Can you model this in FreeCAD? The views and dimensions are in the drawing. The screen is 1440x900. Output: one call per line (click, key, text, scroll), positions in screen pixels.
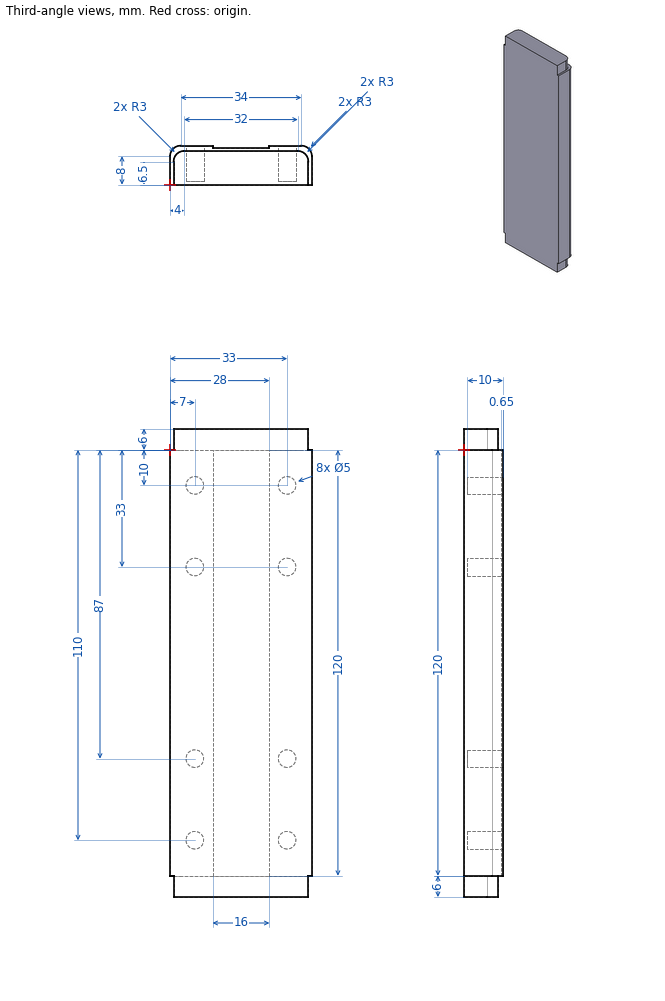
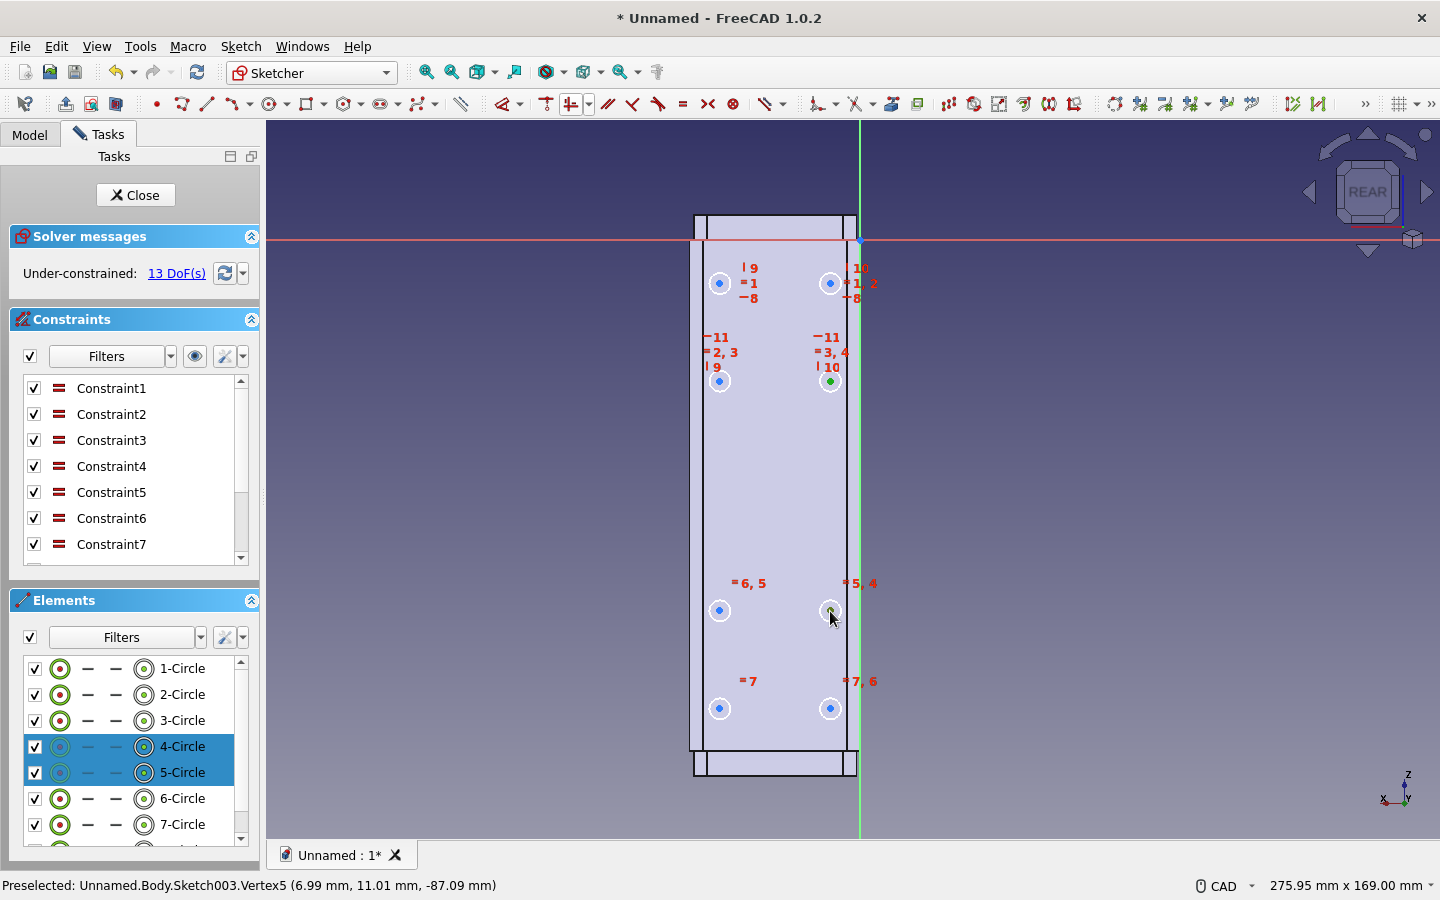
click(588, 104)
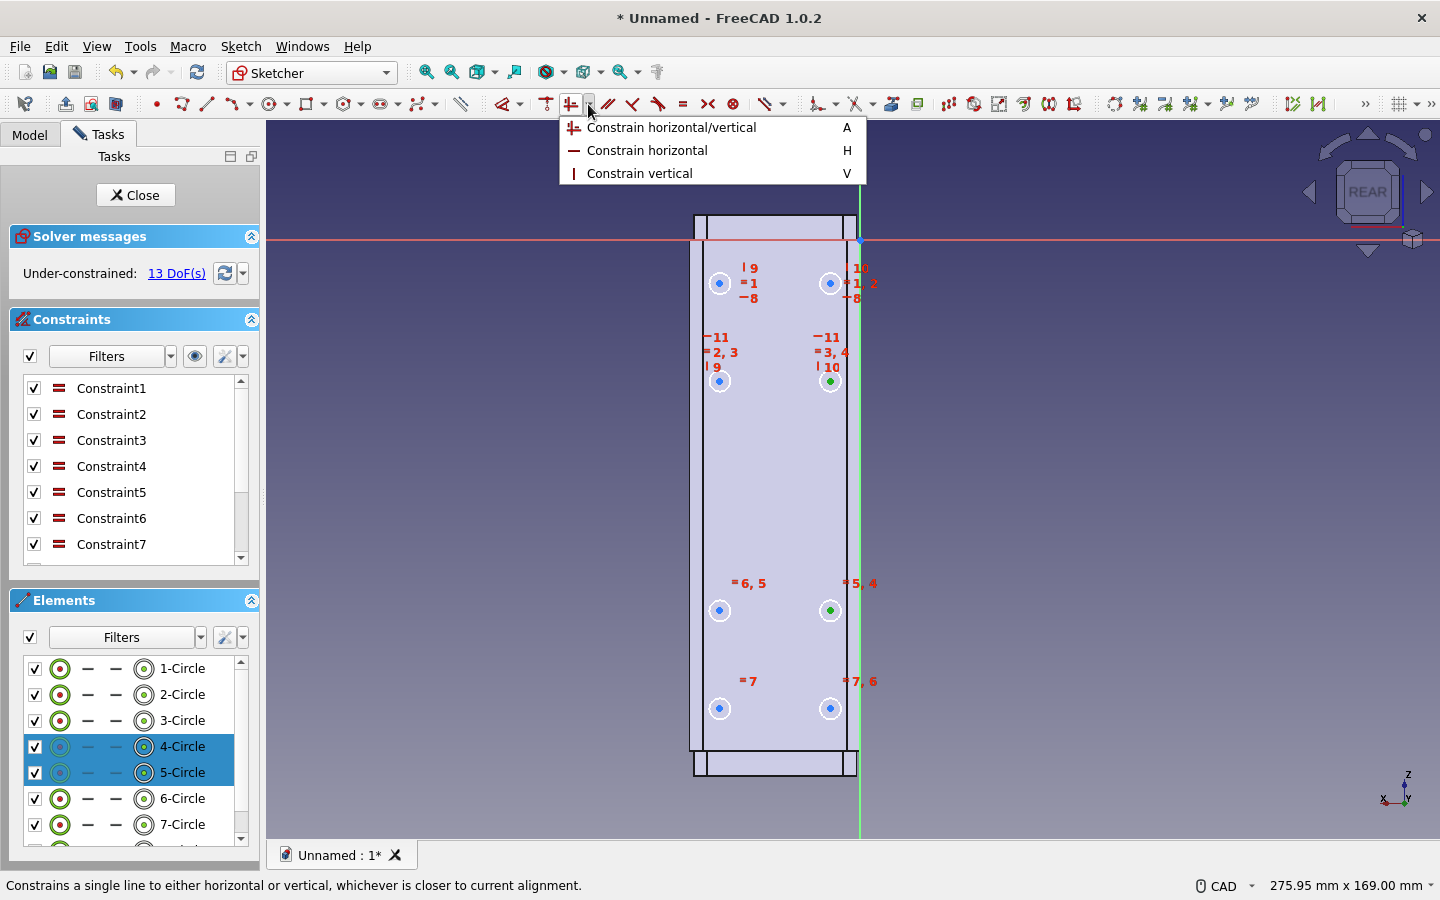
click(713, 174)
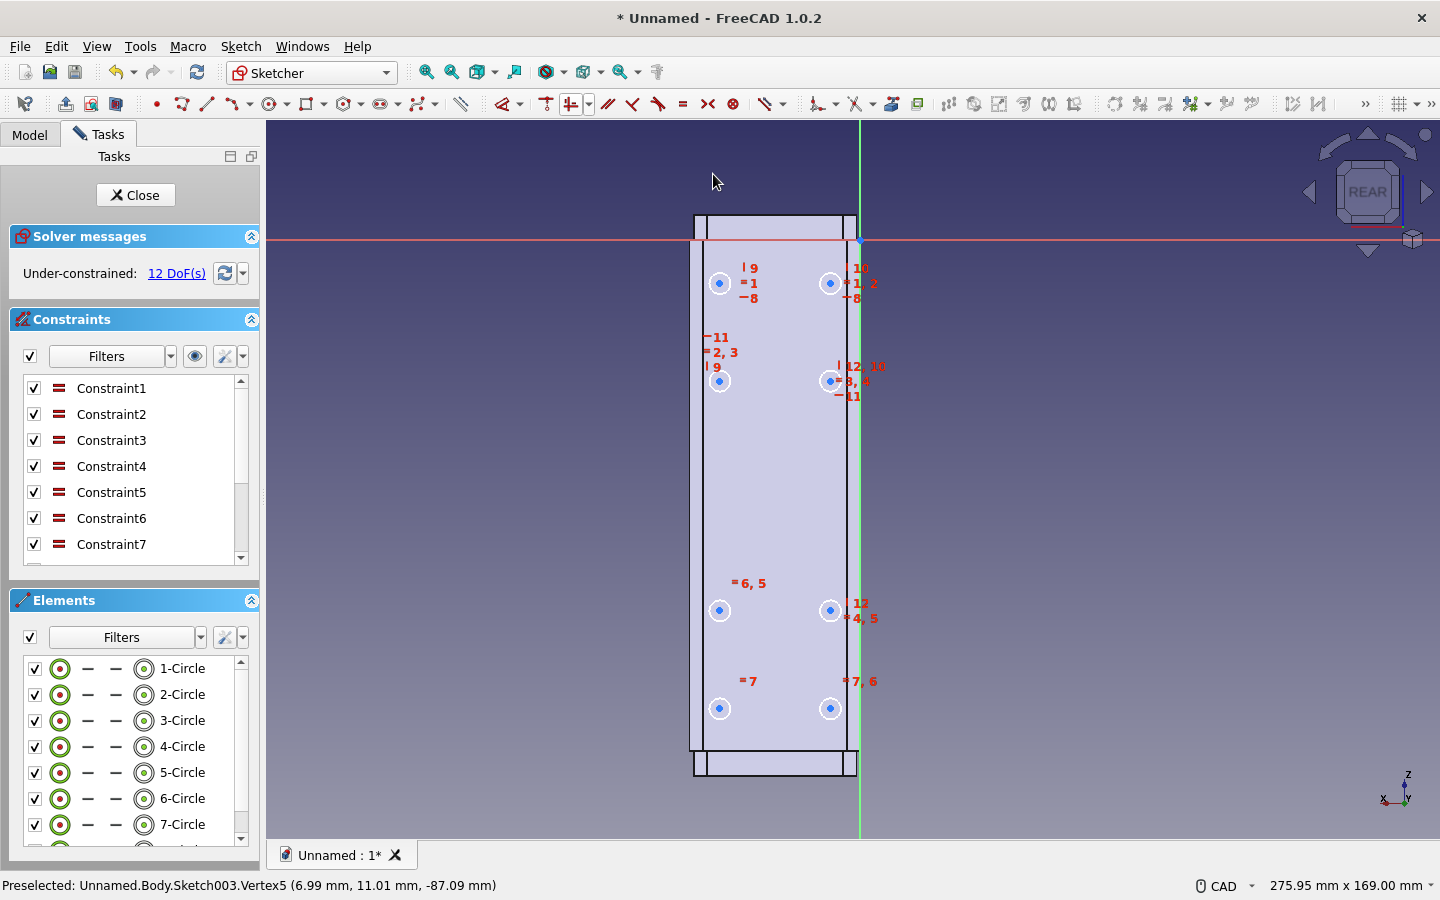
click(720, 381)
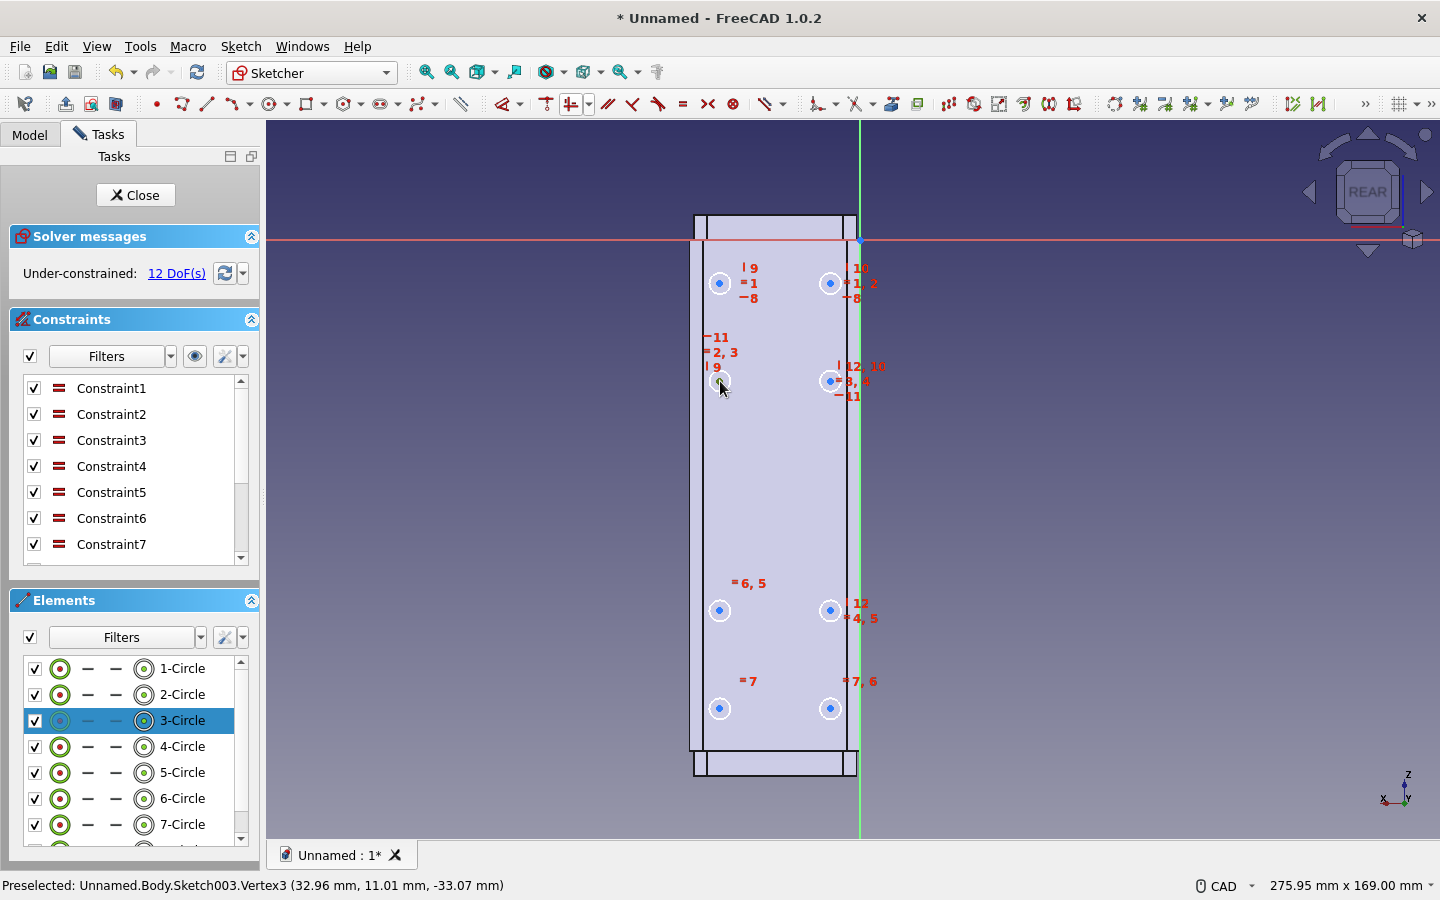
click(720, 611)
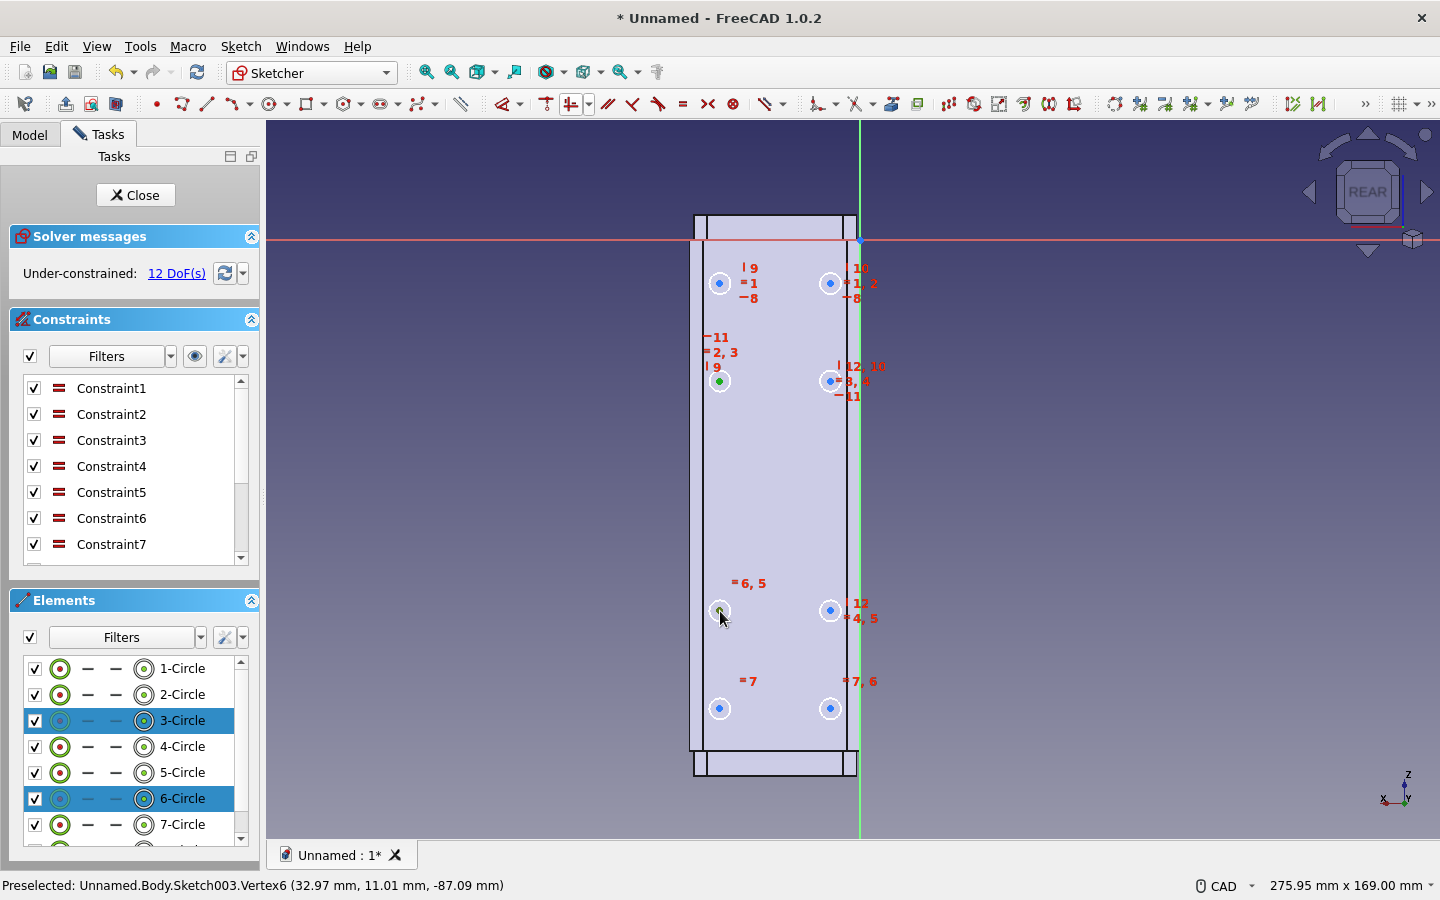
key(v)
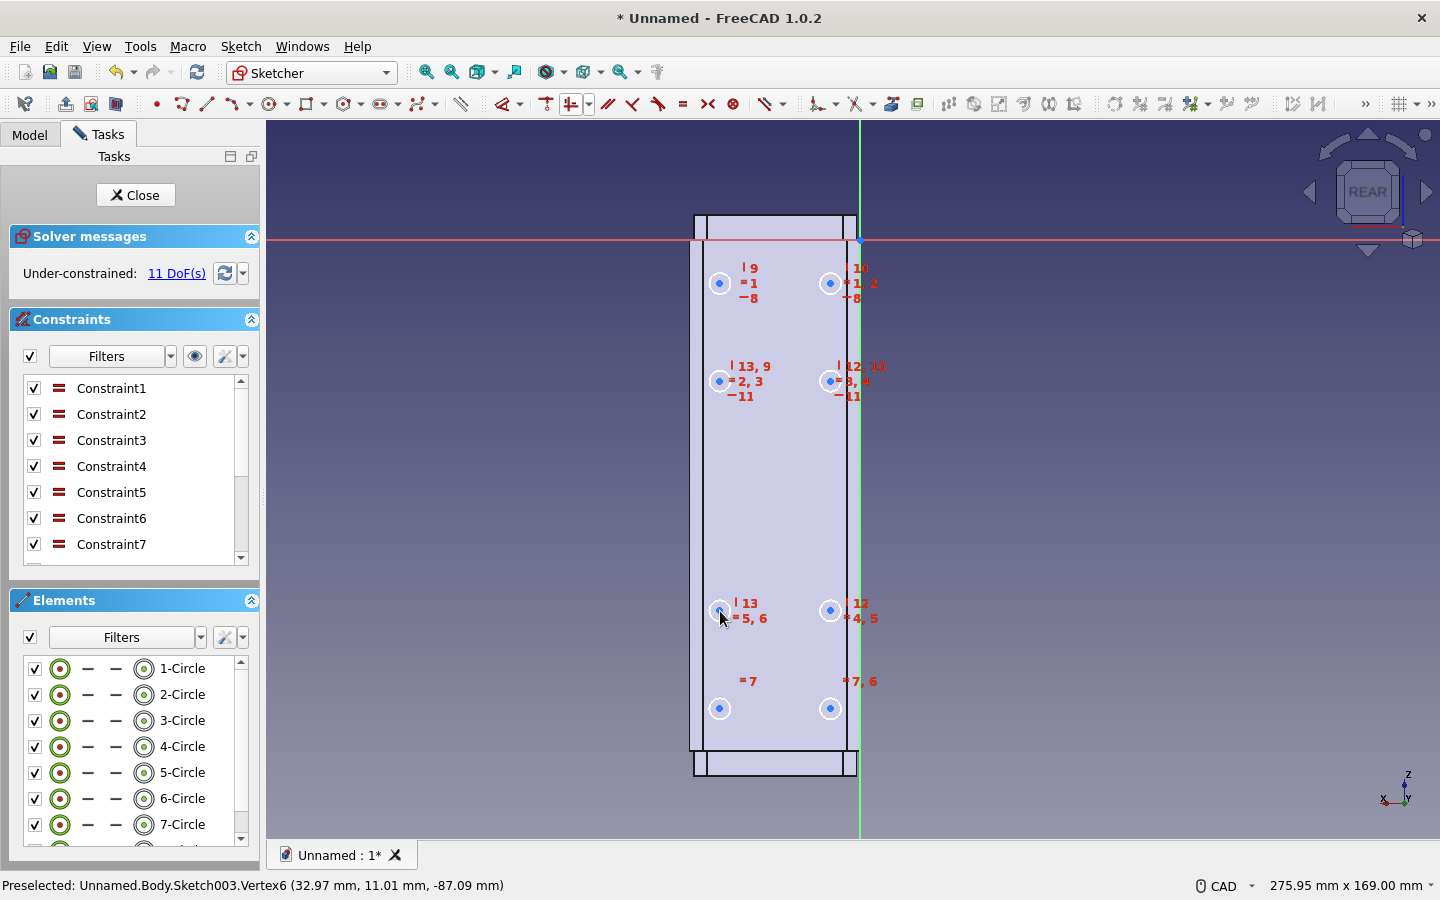
click(831, 611)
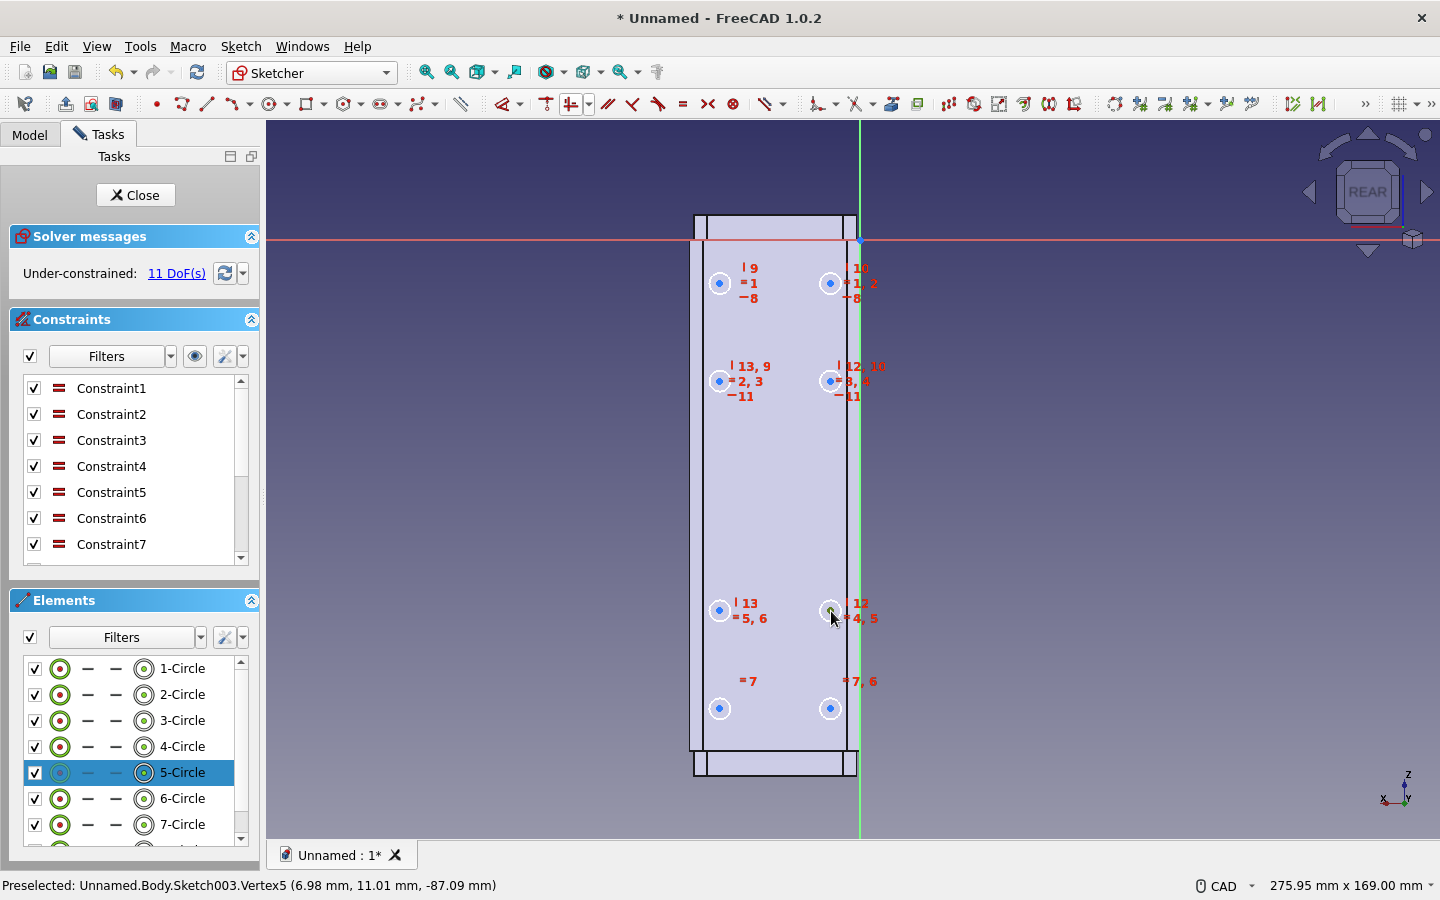
click(720, 611)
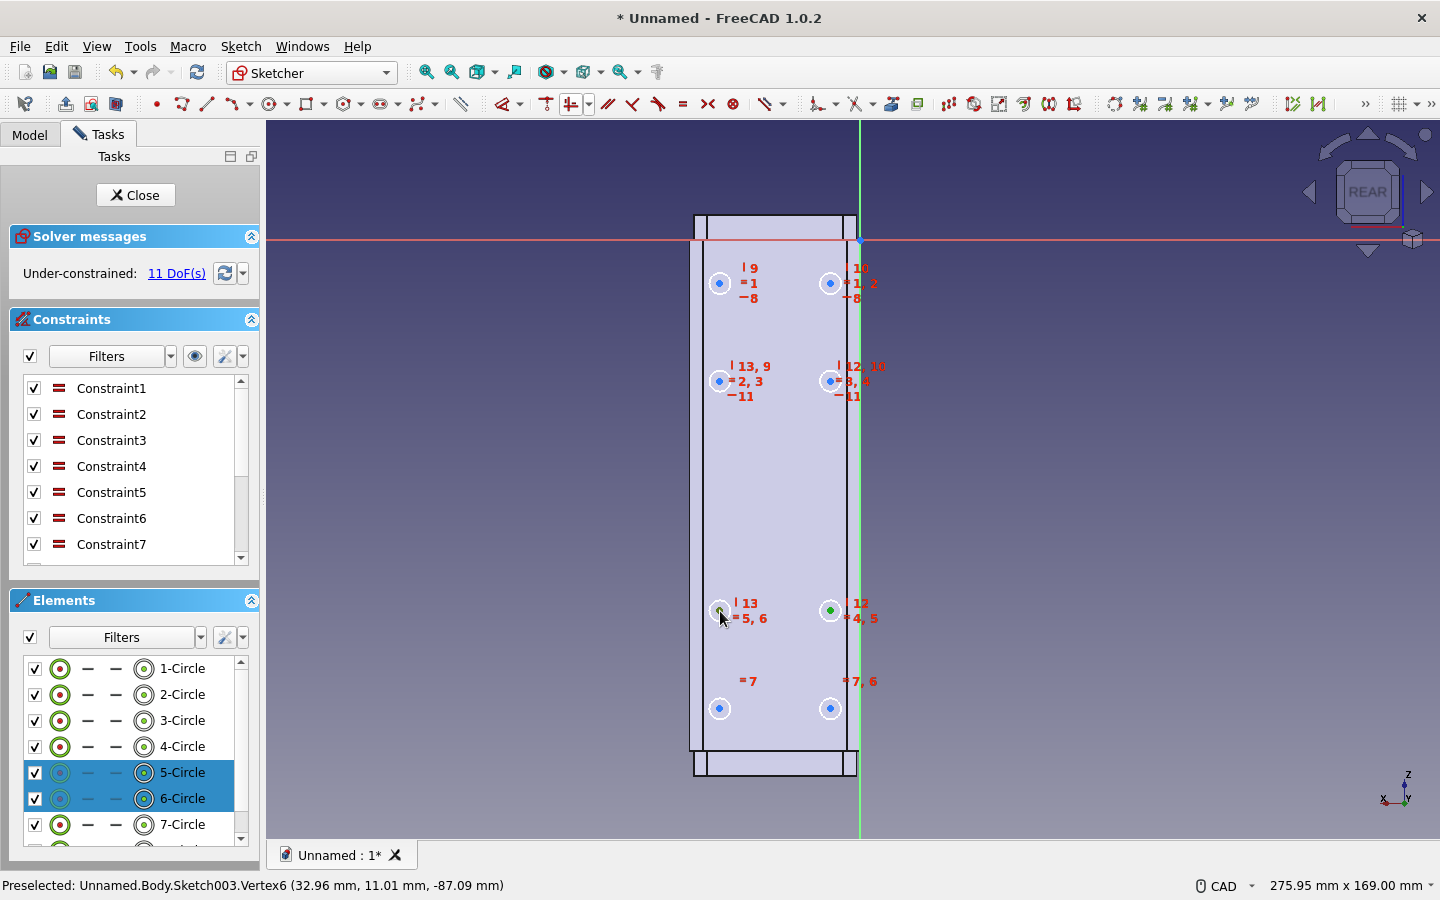
click(588, 104)